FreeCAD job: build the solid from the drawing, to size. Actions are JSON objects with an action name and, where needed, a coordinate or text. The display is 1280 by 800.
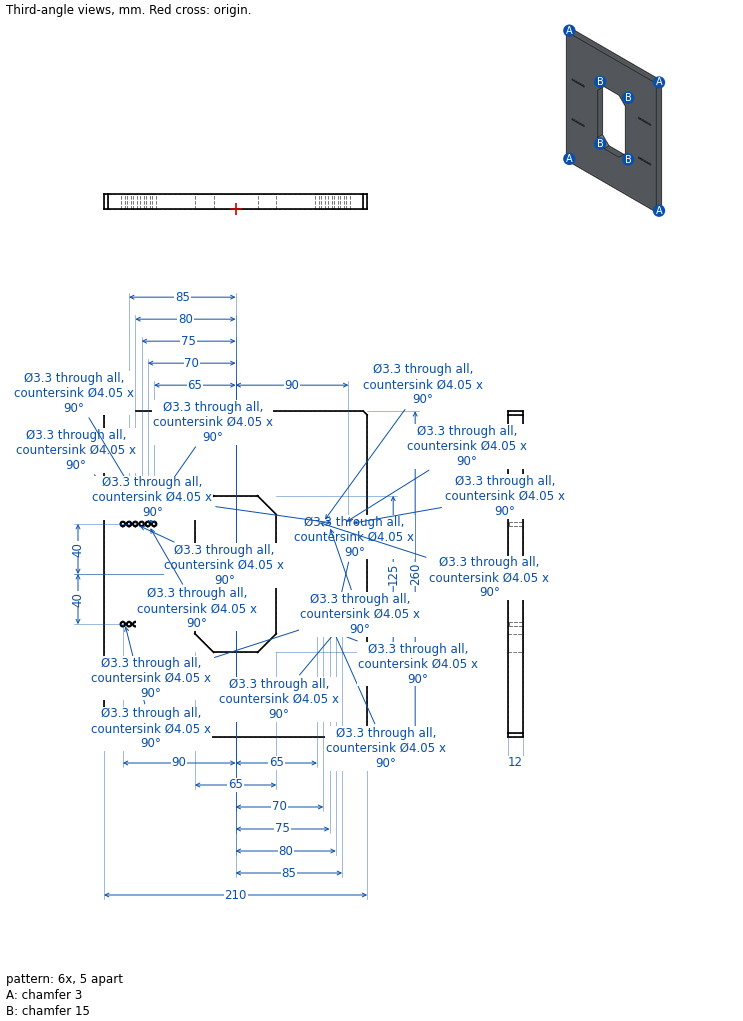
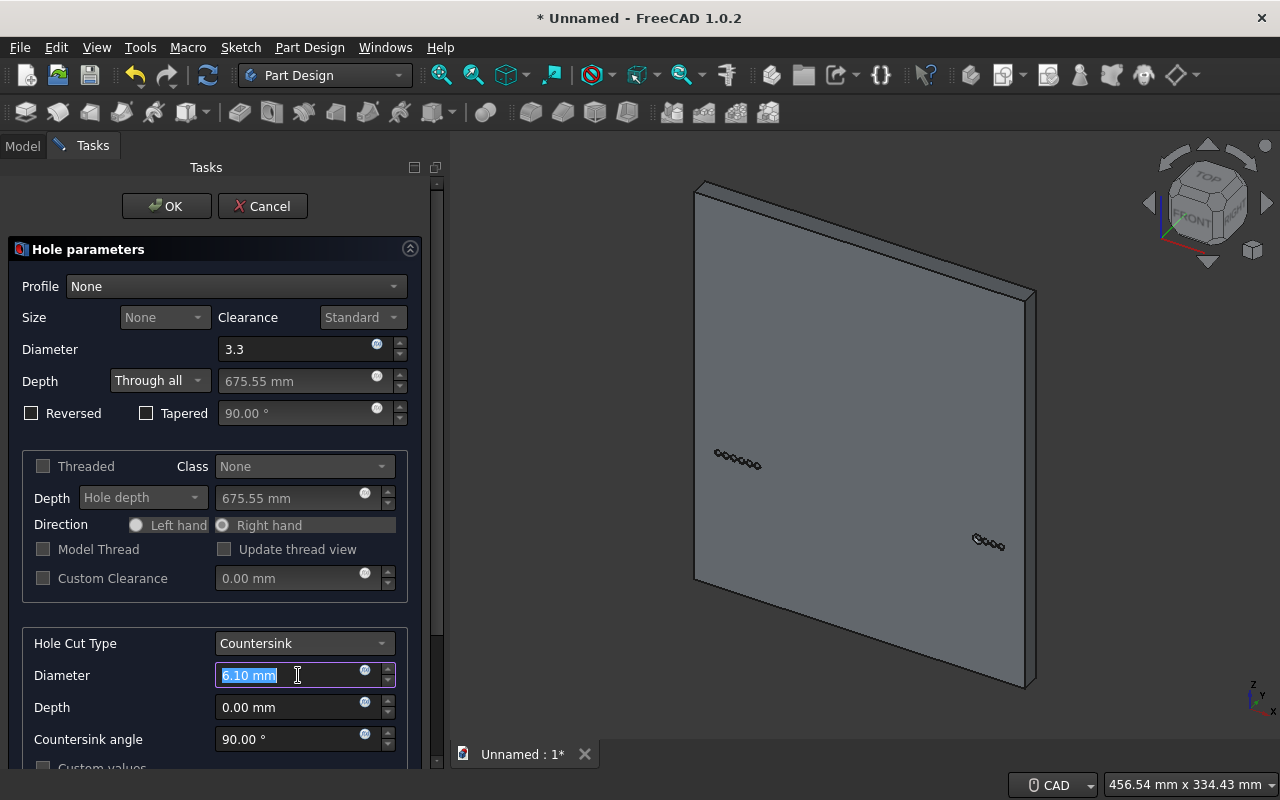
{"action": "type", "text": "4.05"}
{"action": "key", "text": "Tab"}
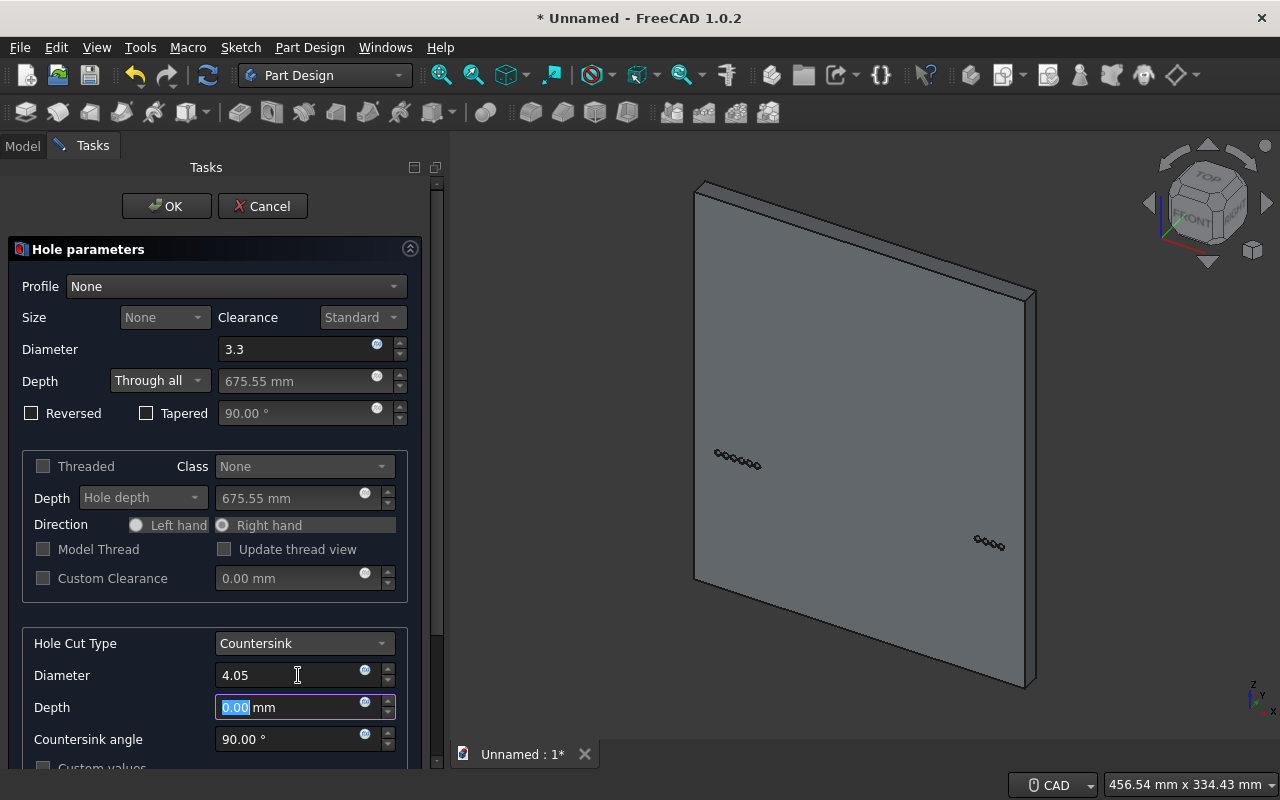
{"action": "left_click", "coordinate": [167, 206]}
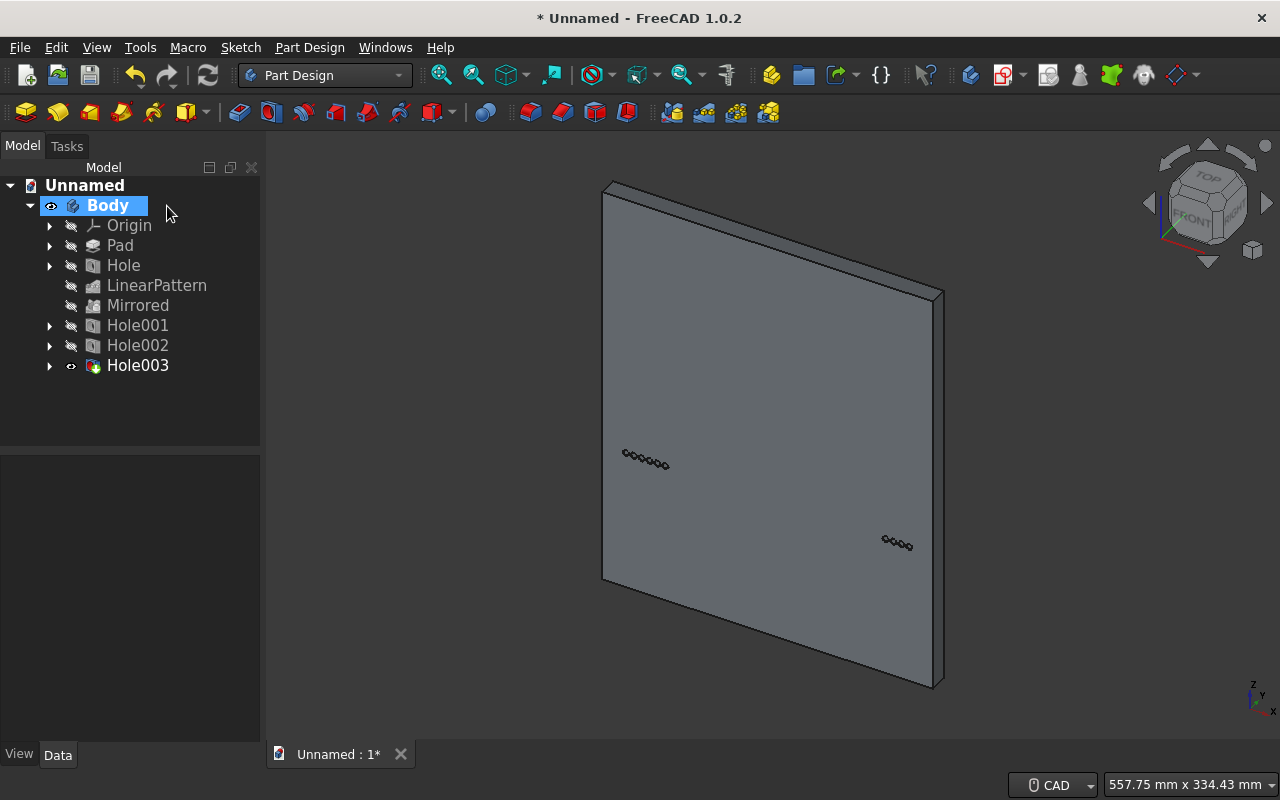
{"action": "left_click", "coordinate": [768, 384]}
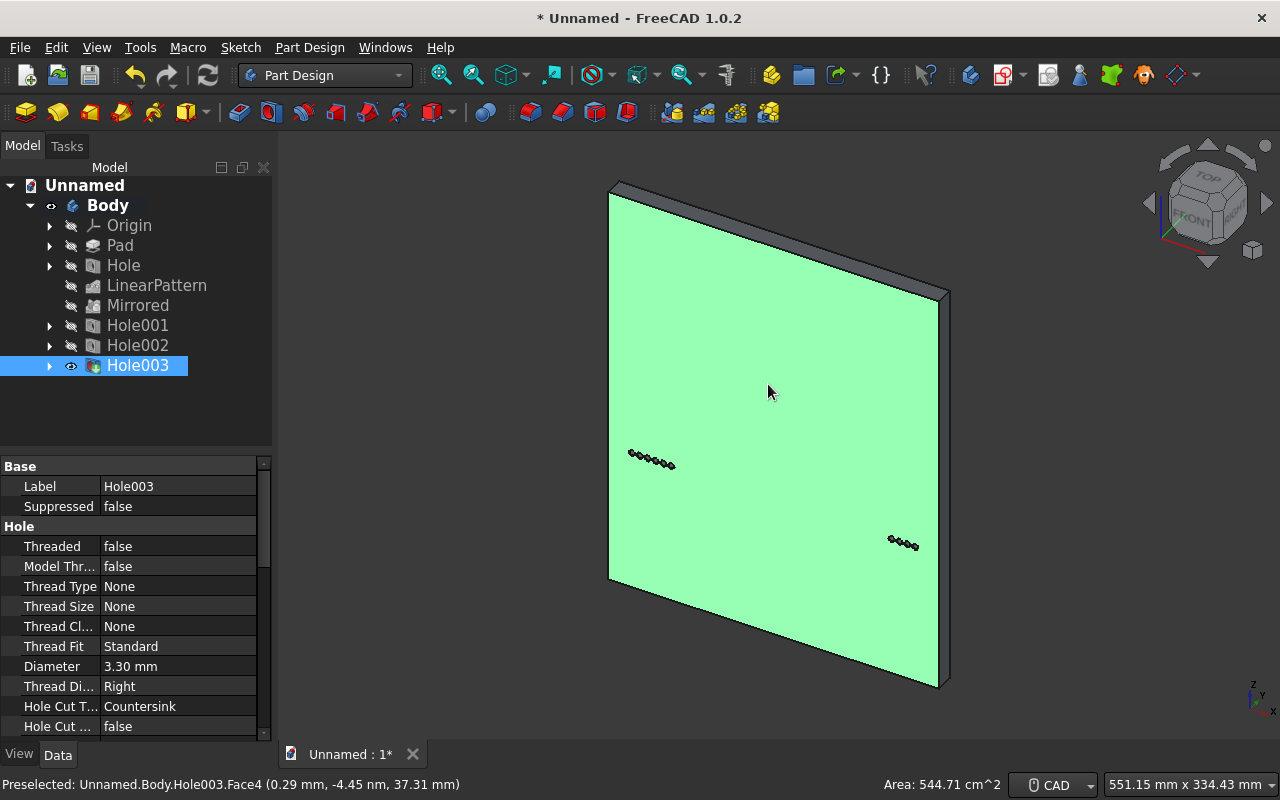
{"action": "left_click", "coordinate": [1004, 76]}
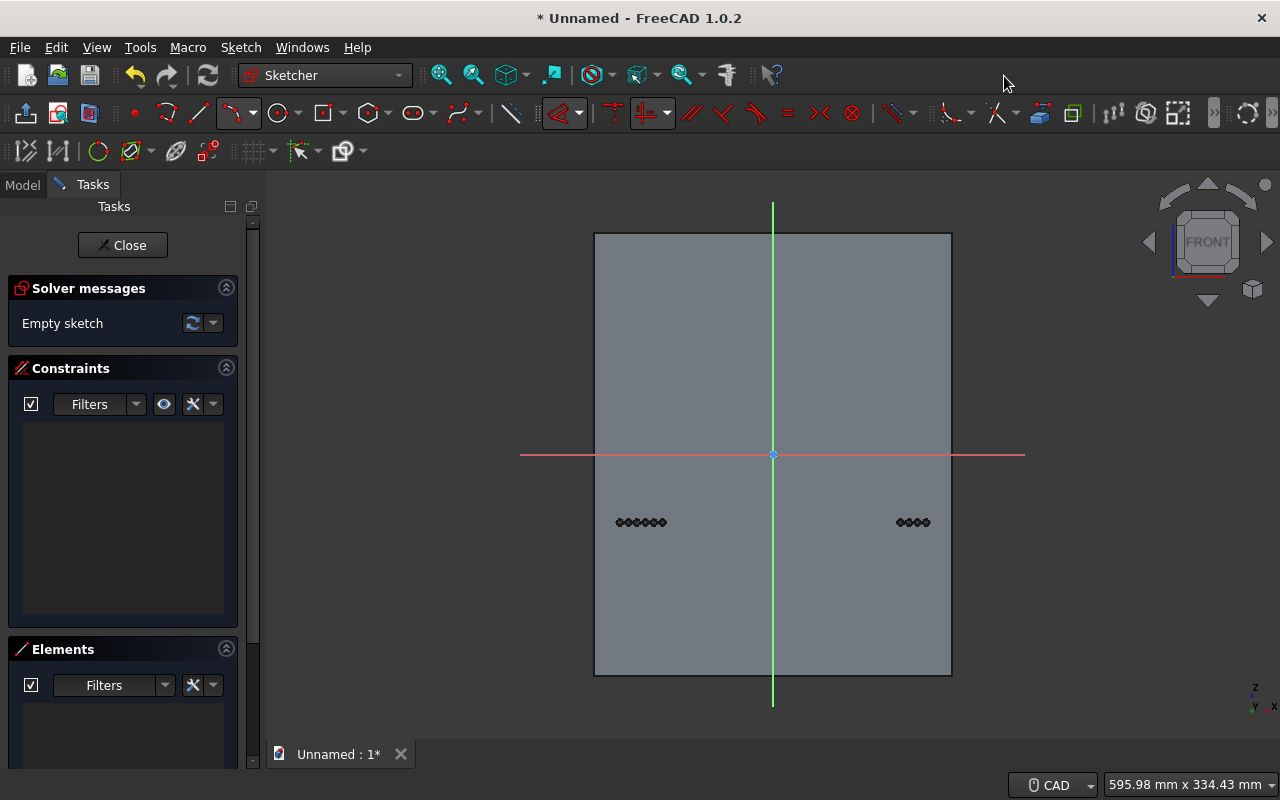
{"action": "scroll", "coordinate": [902, 526], "scroll_direction": "up", "scroll_amount": 15}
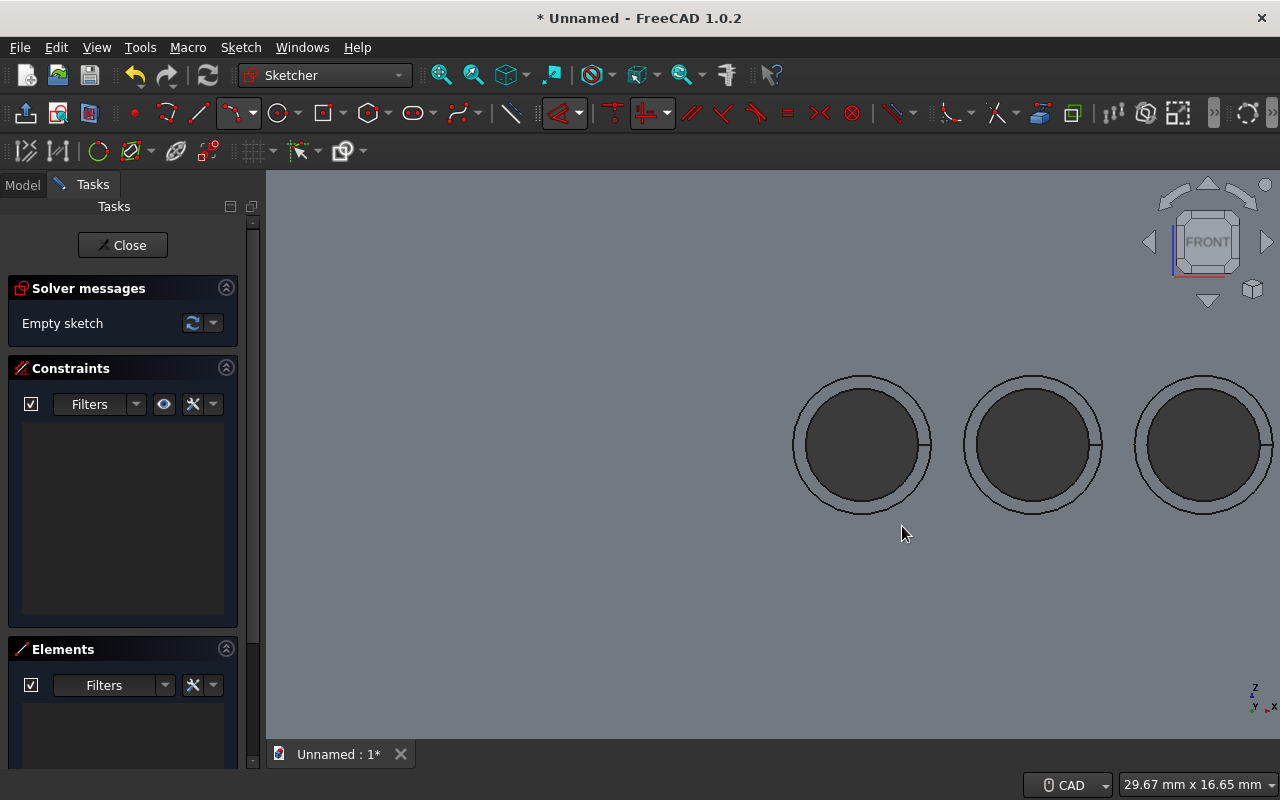
{"action": "scroll", "coordinate": [685, 441], "scroll_direction": "up", "scroll_amount": 6}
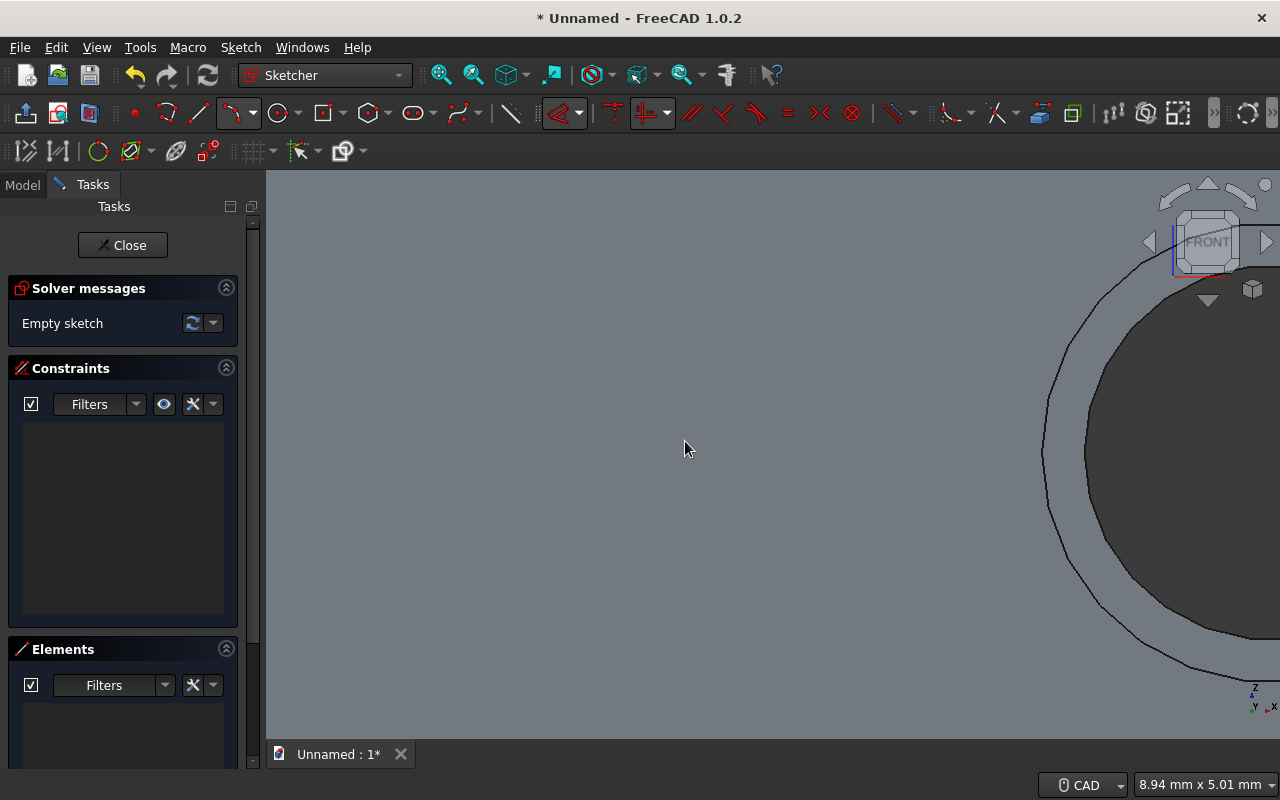
{"action": "left_click", "coordinate": [278, 114]}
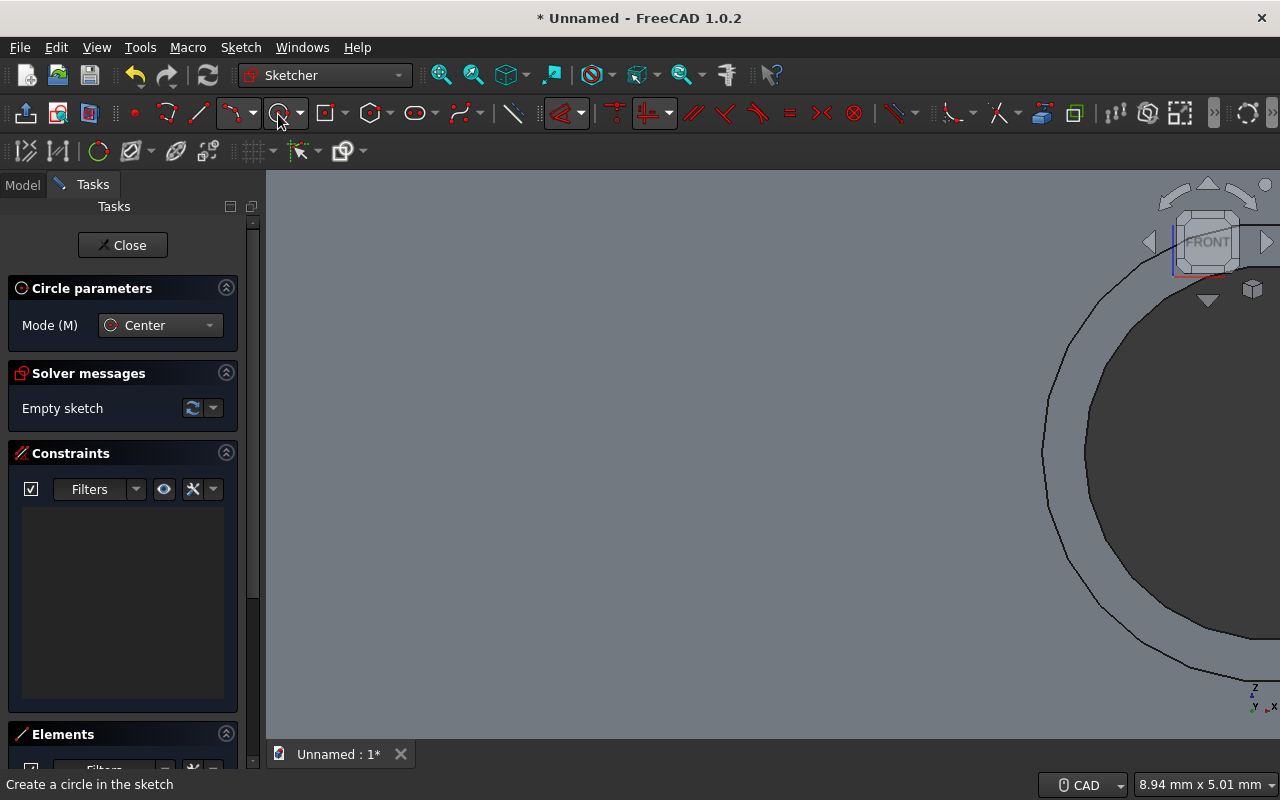
{"action": "left_click", "coordinate": [704, 453]}
{"action": "mouse_move", "coordinate": [837, 320]}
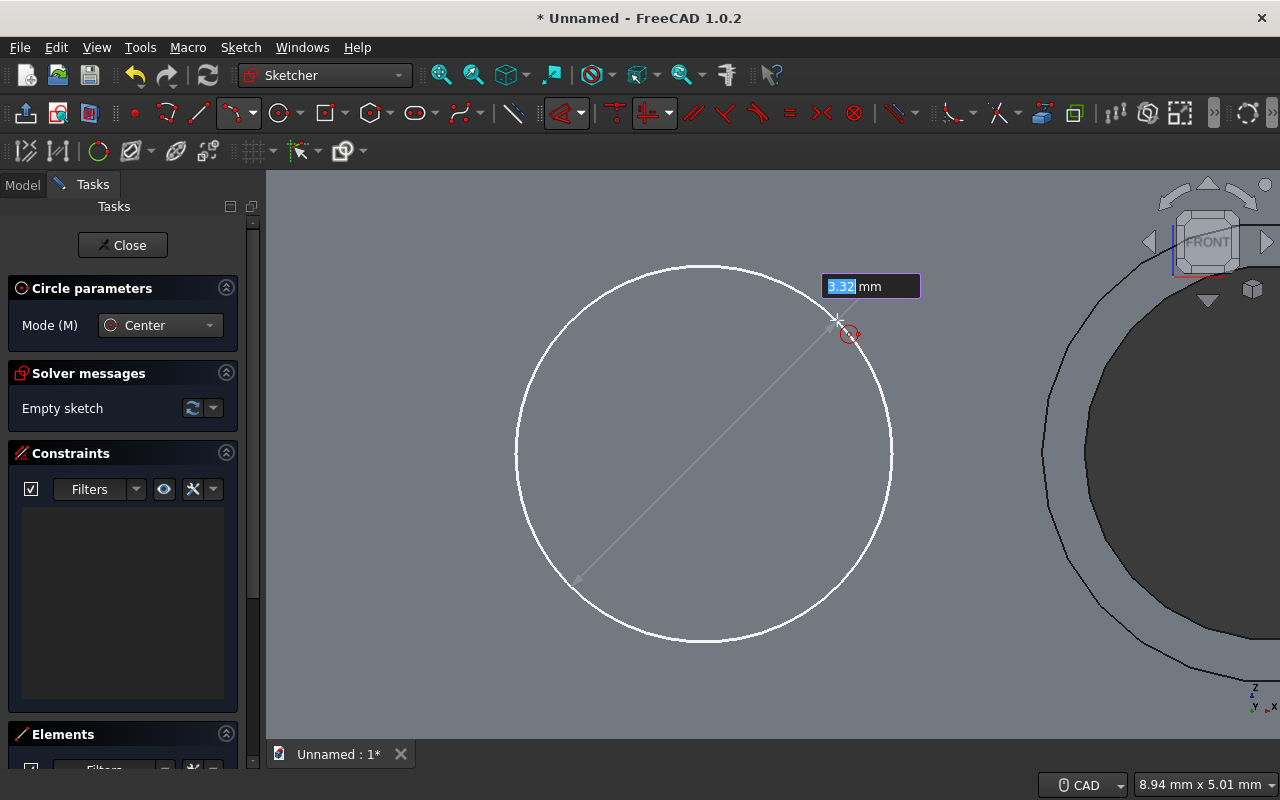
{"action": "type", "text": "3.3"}
{"action": "key", "text": "Return"}
{"action": "key", "text": "Escape"}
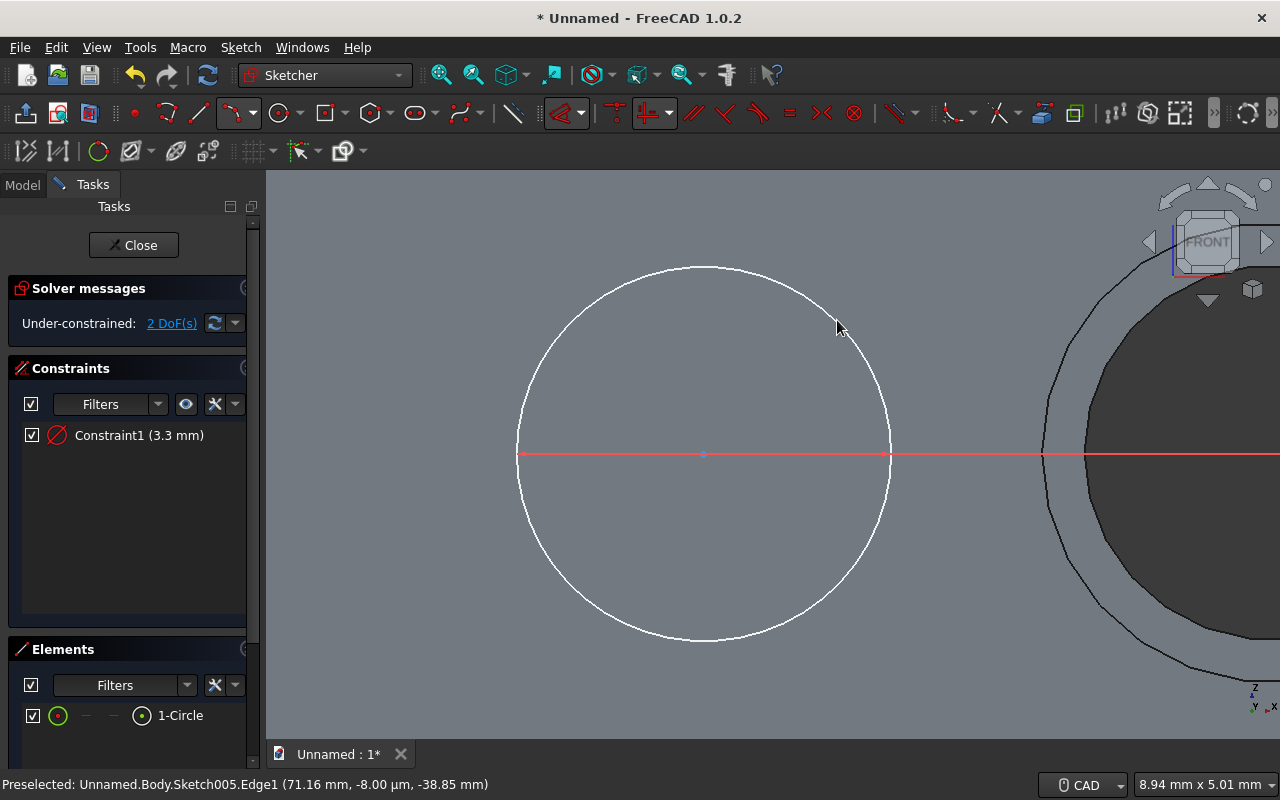
{"action": "left_click", "coordinate": [704, 454]}